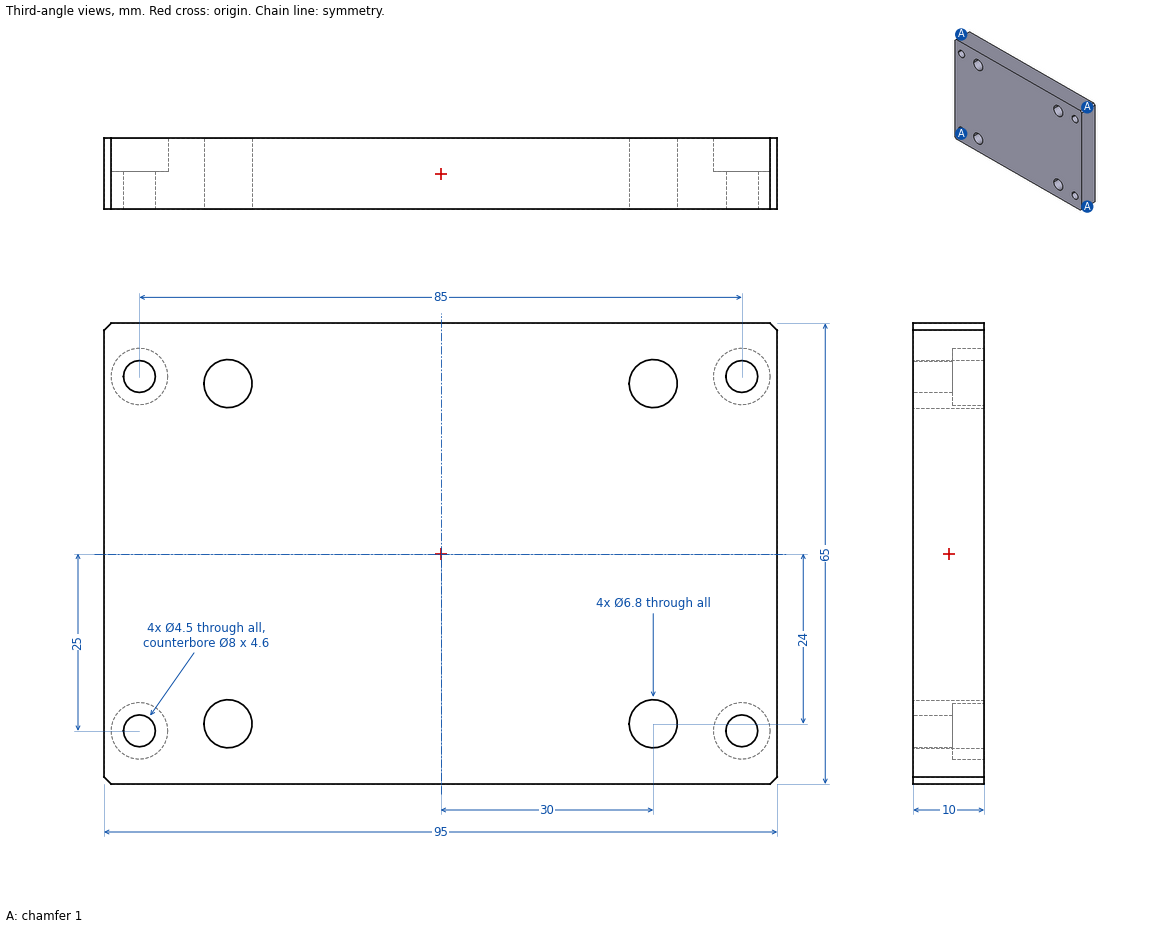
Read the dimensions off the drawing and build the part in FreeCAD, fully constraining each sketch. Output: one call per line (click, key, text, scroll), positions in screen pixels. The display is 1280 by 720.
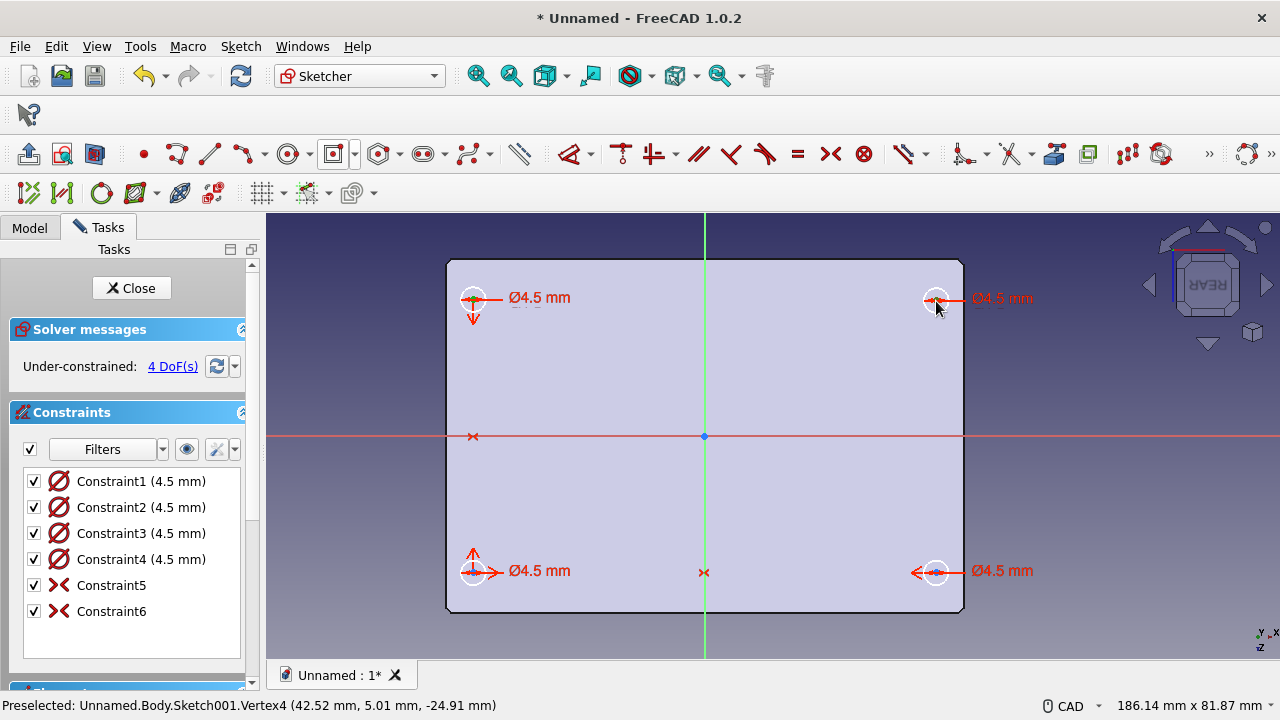
click(705, 603)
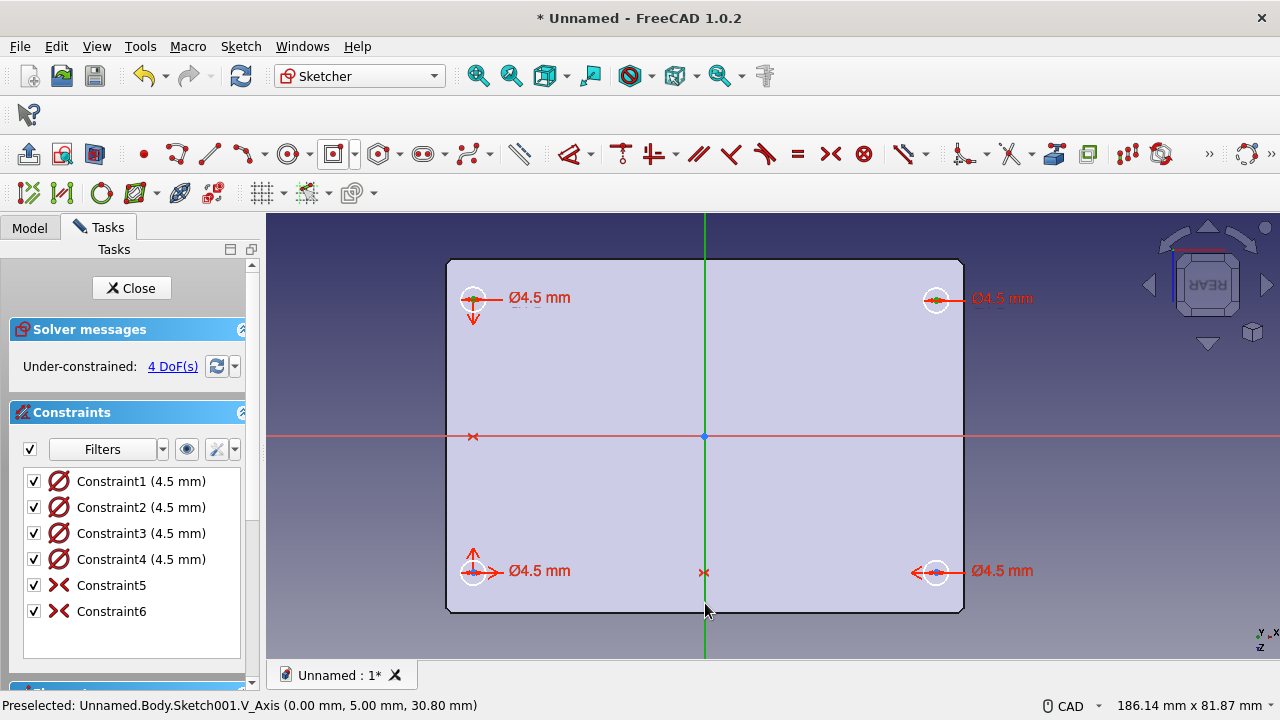
key(s)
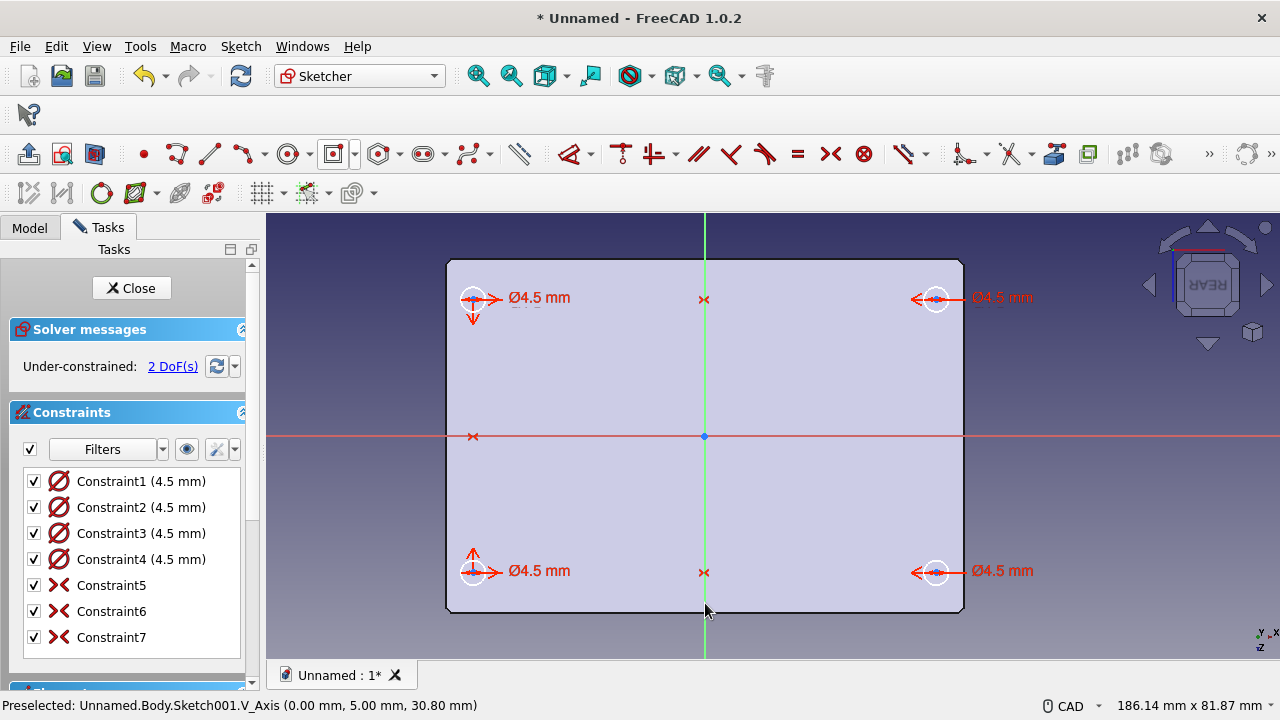
click(568, 154)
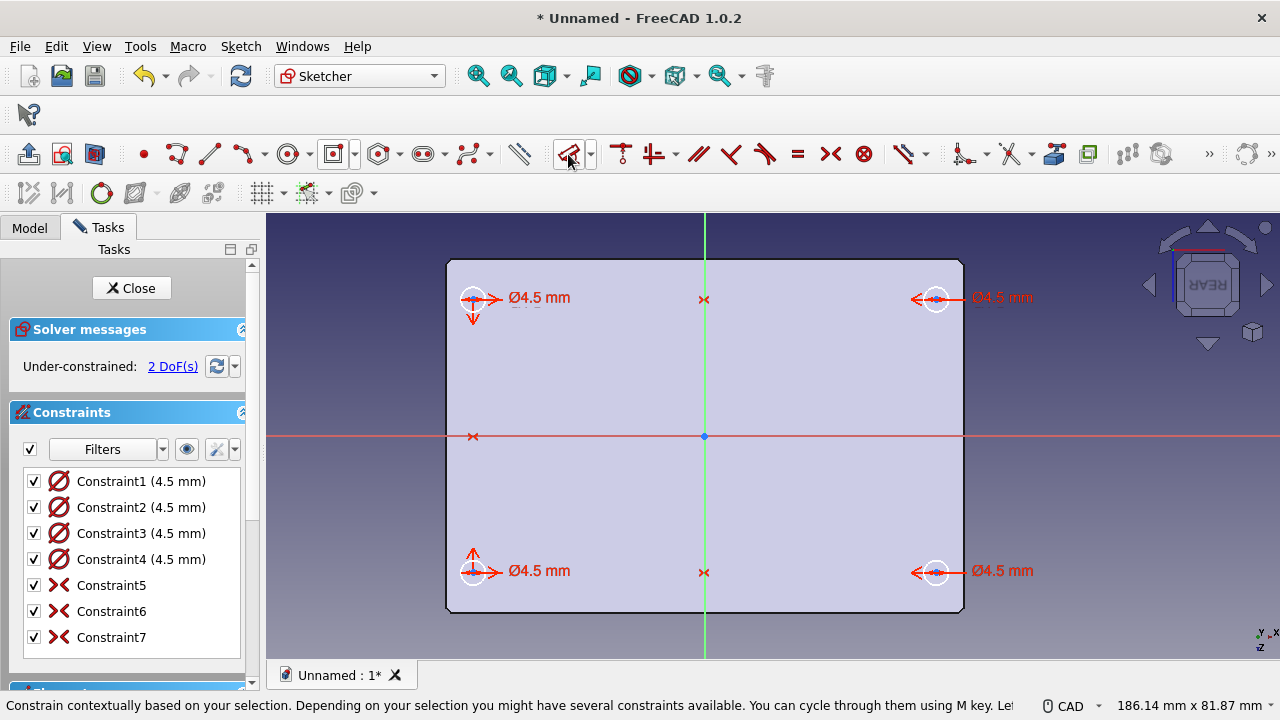
click(473, 300)
click(439, 368)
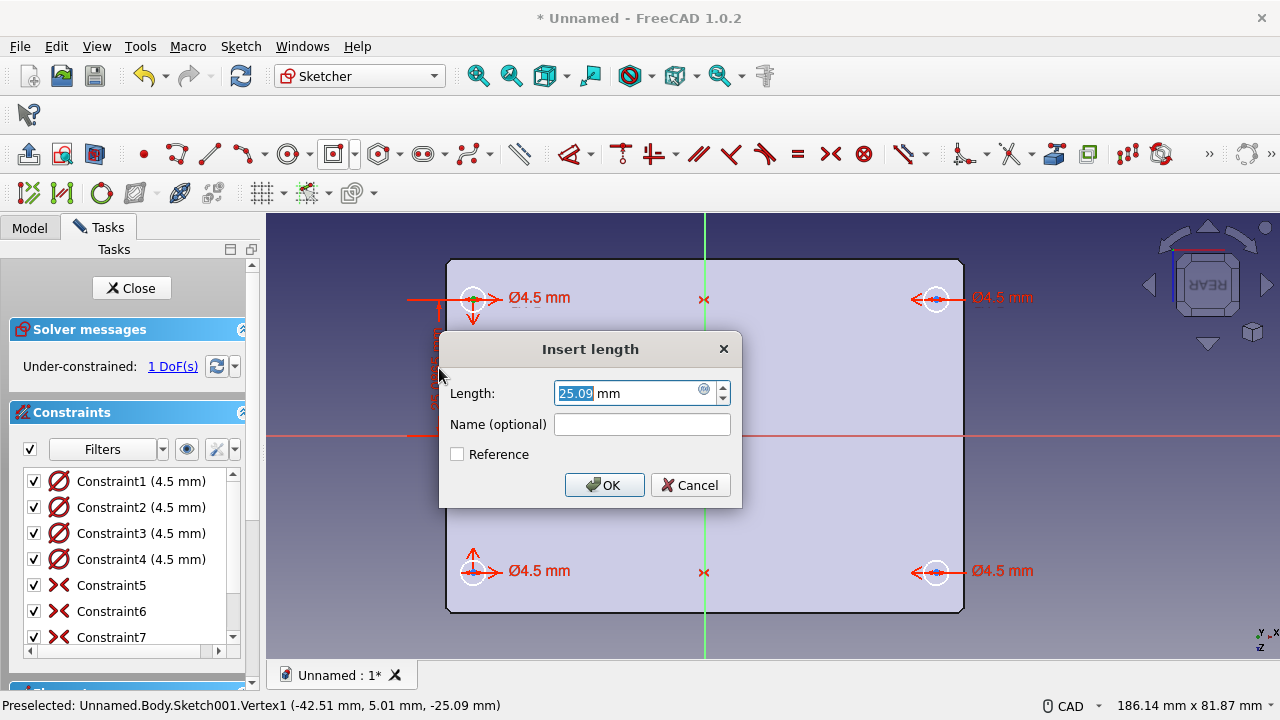
text(25)
key(Return)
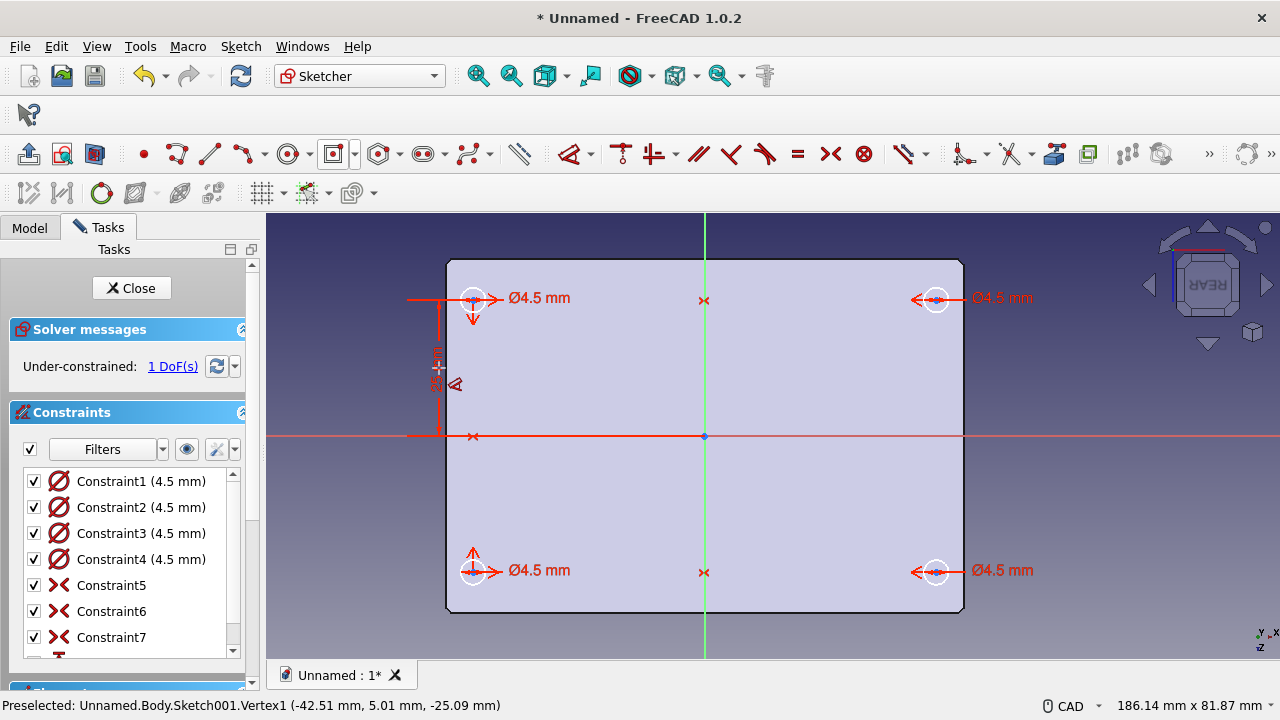
click(473, 572)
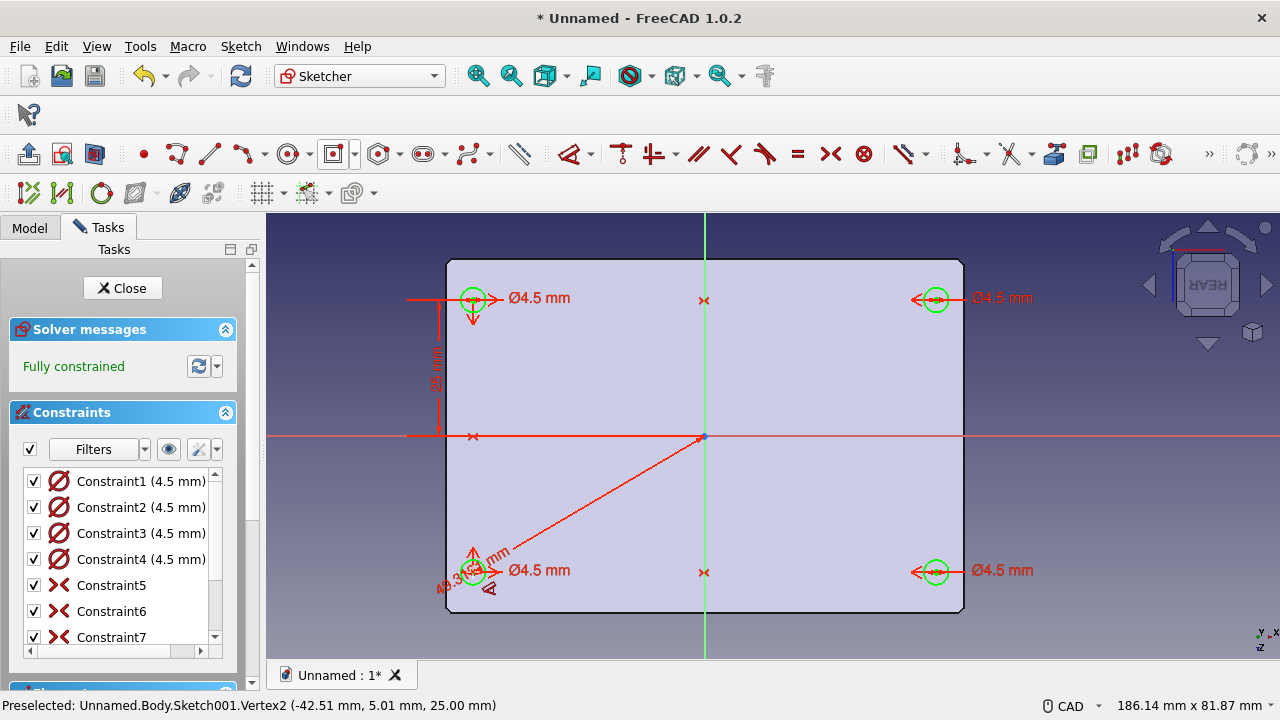
click(936, 572)
click(598, 606)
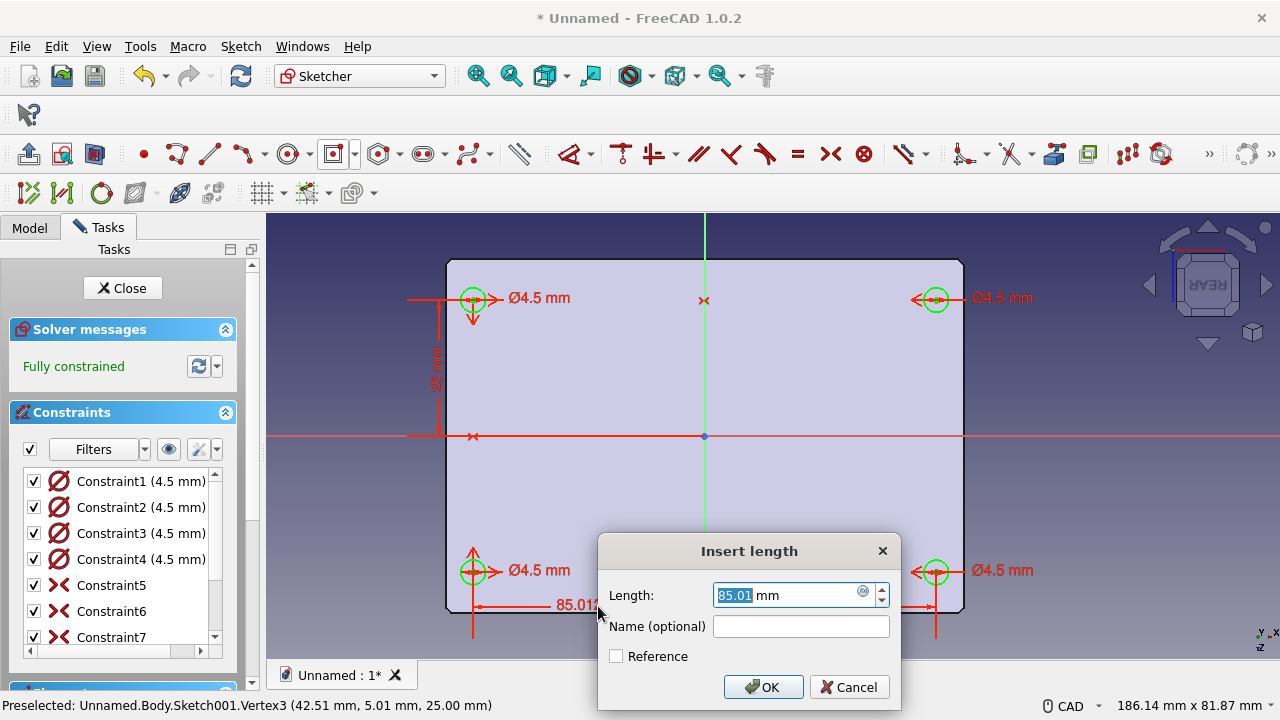
text(85)
key(Return)
key(Escape)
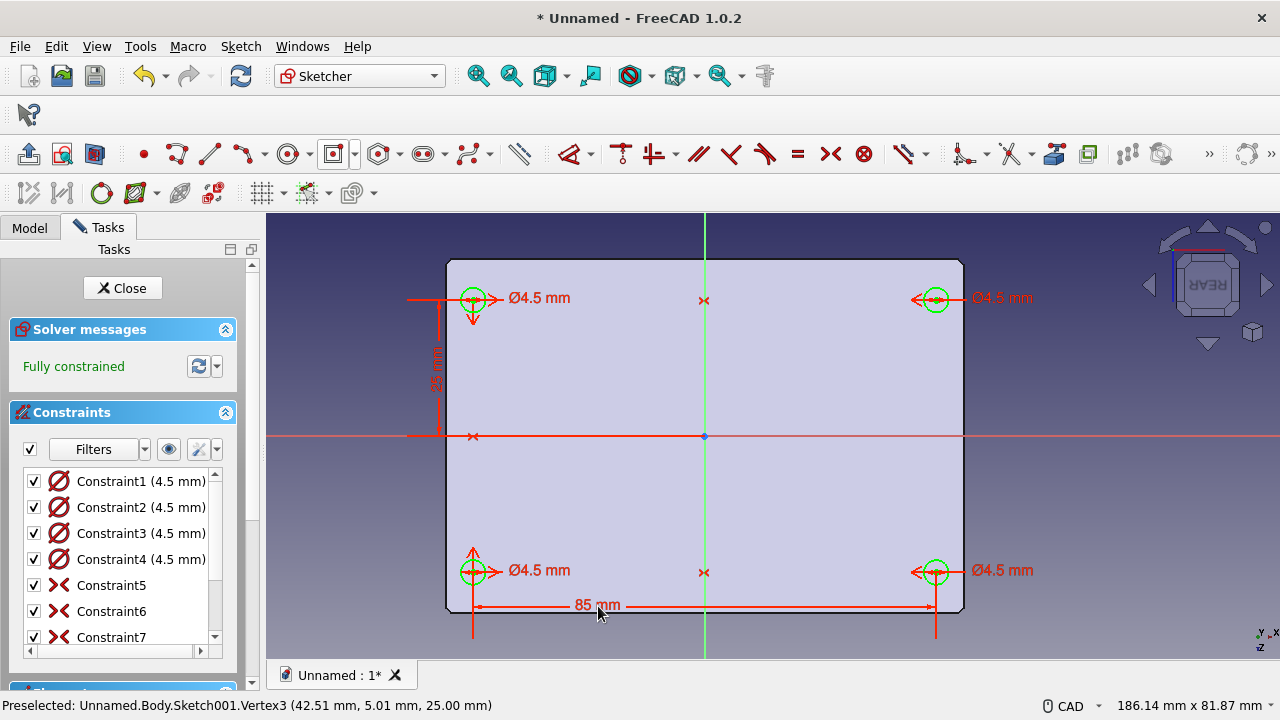
click(123, 288)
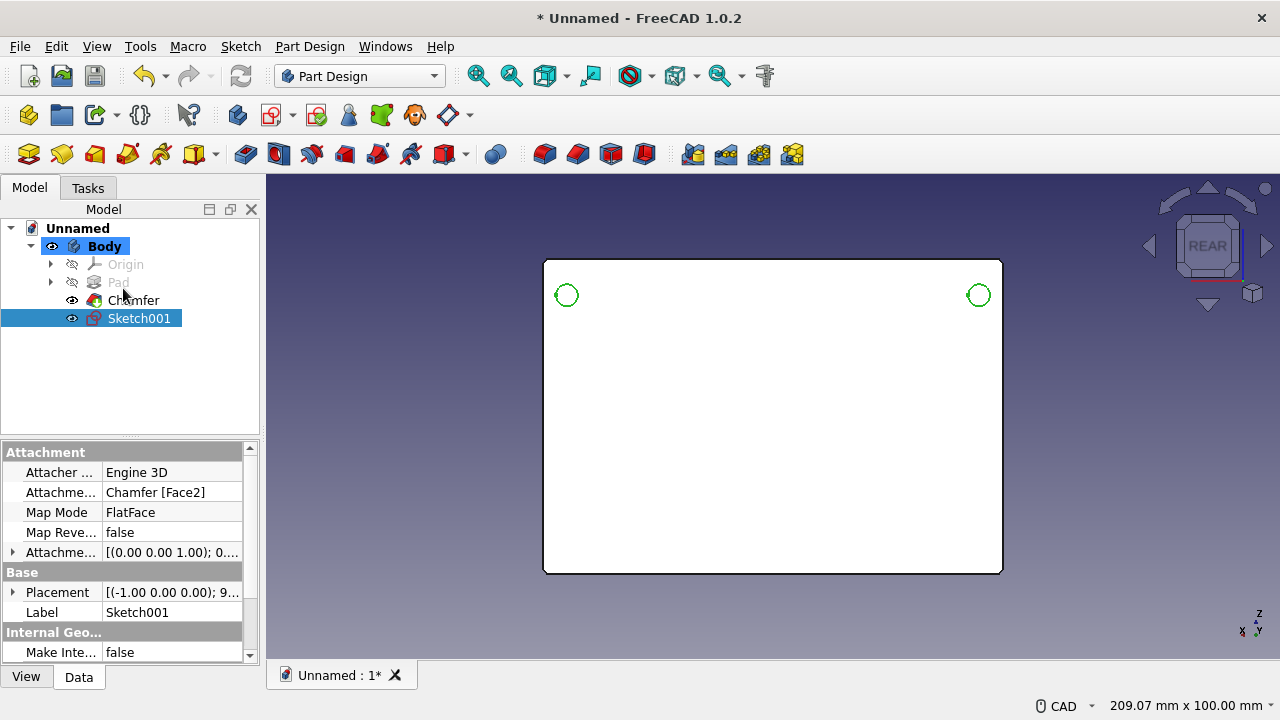
click(279, 154)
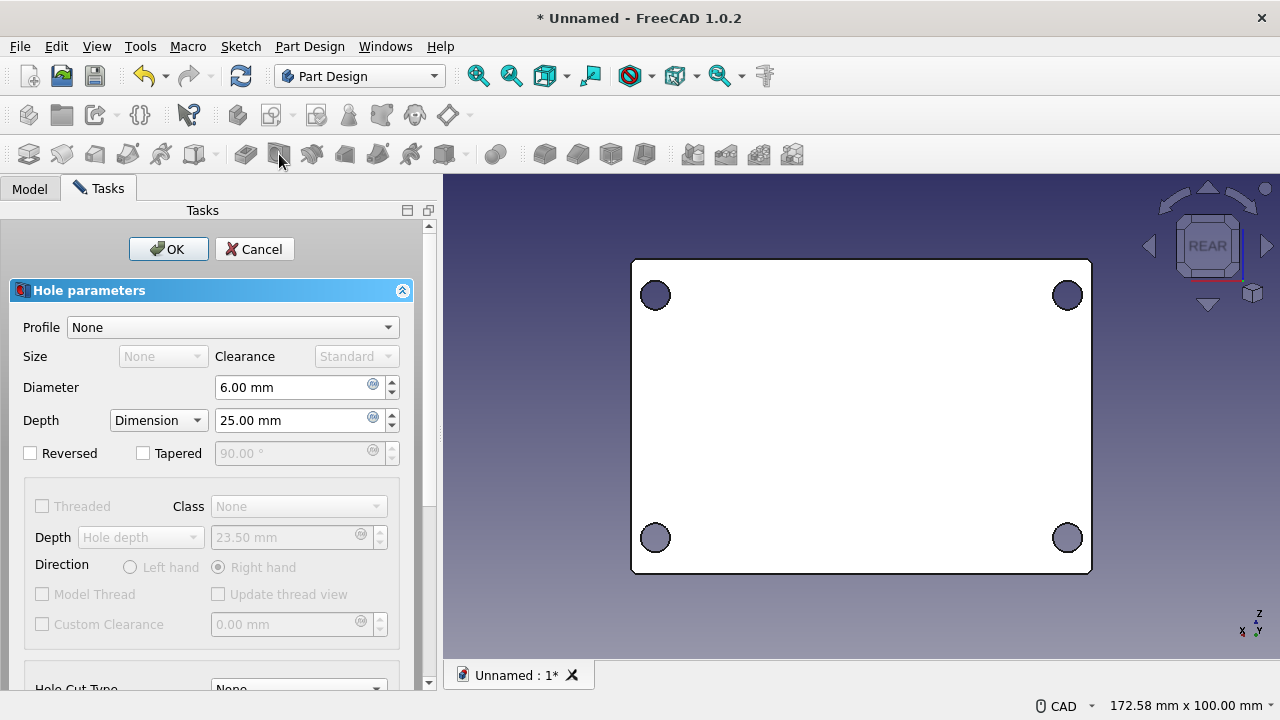
triple_click(300, 388)